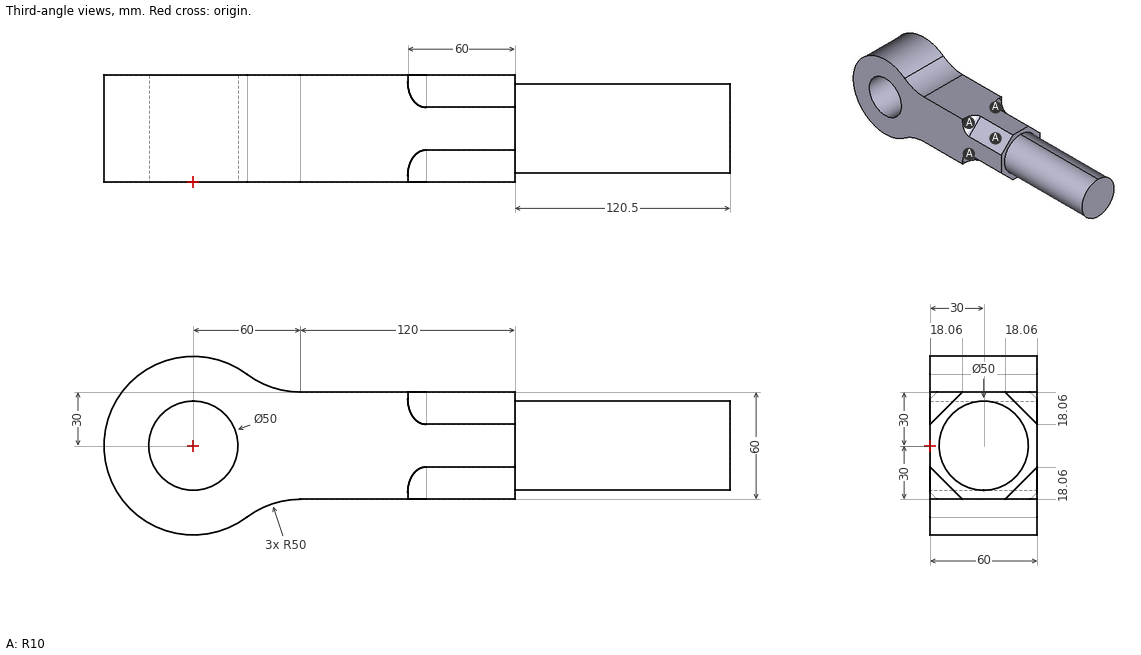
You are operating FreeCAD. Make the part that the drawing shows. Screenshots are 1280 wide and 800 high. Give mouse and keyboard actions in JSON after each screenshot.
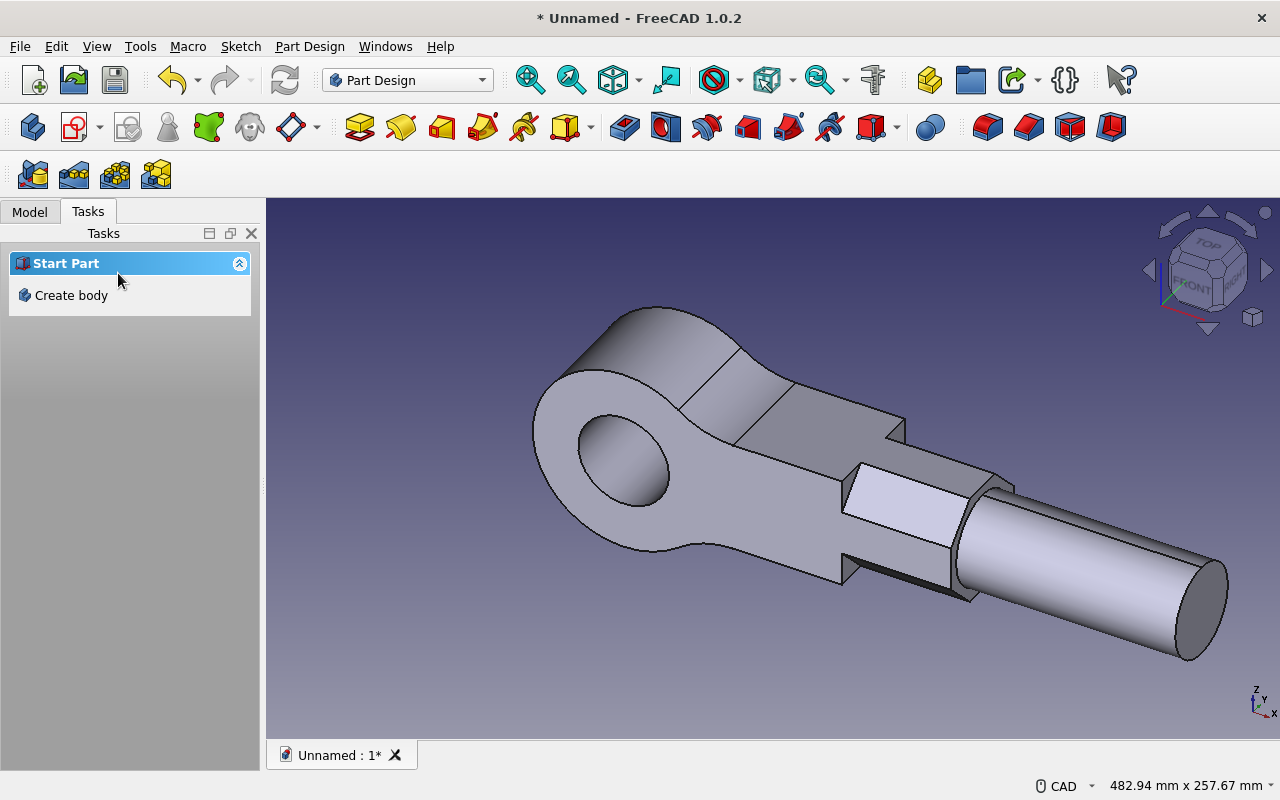
{"action": "key", "text": "0"}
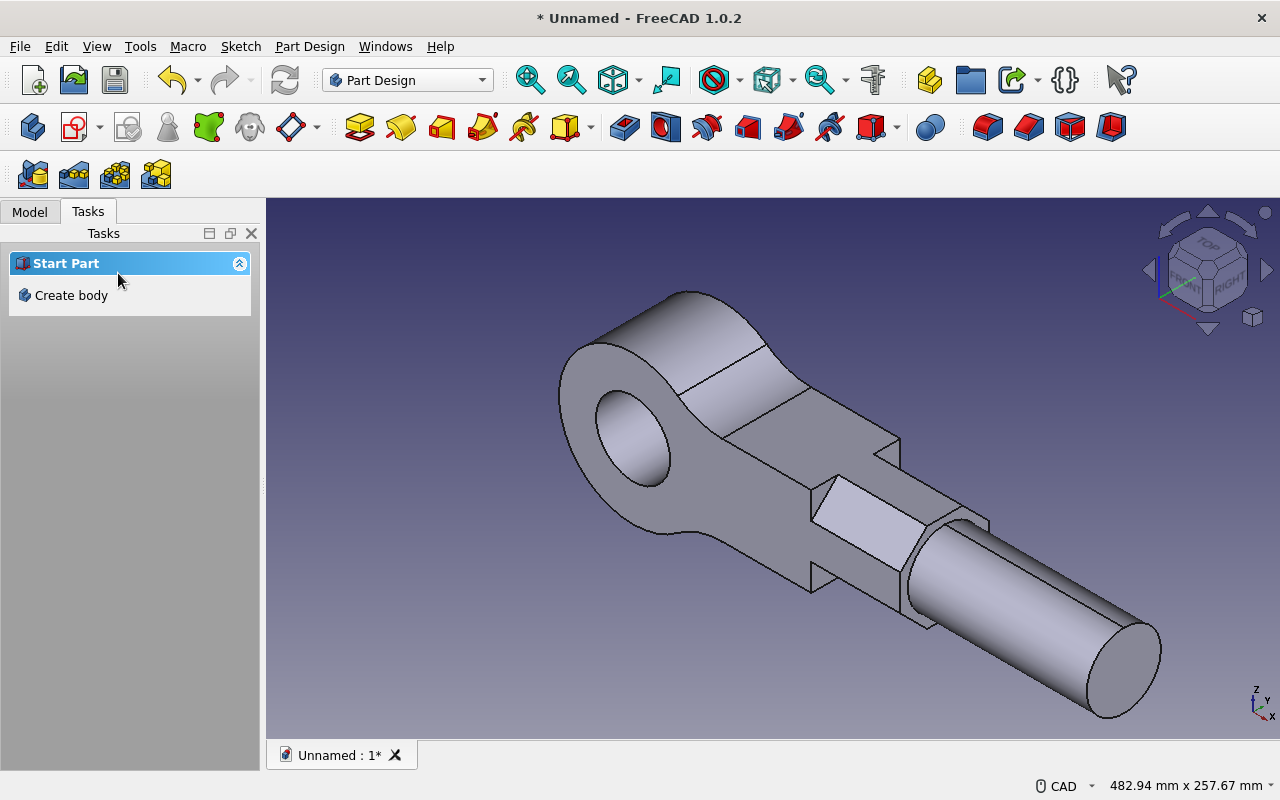
{"action": "key", "text": "v f"}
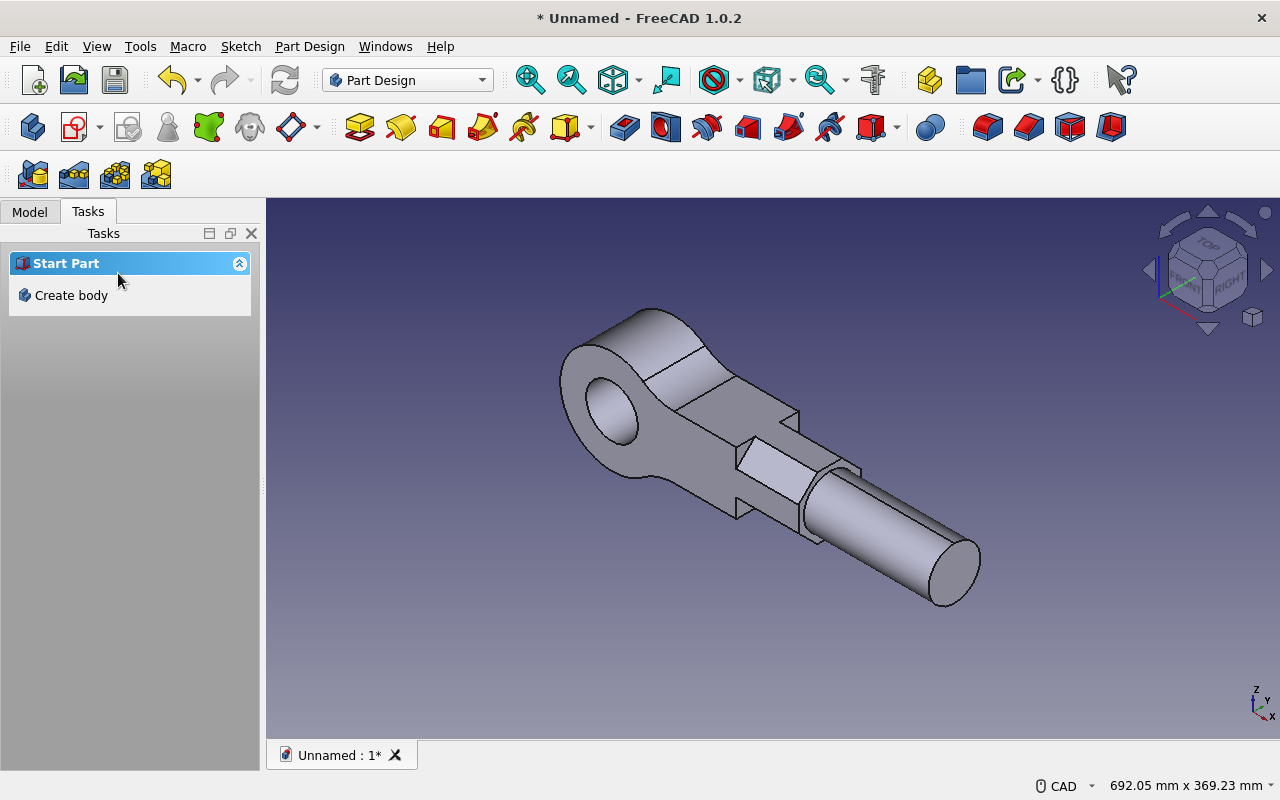
{"action": "key", "text": "2"}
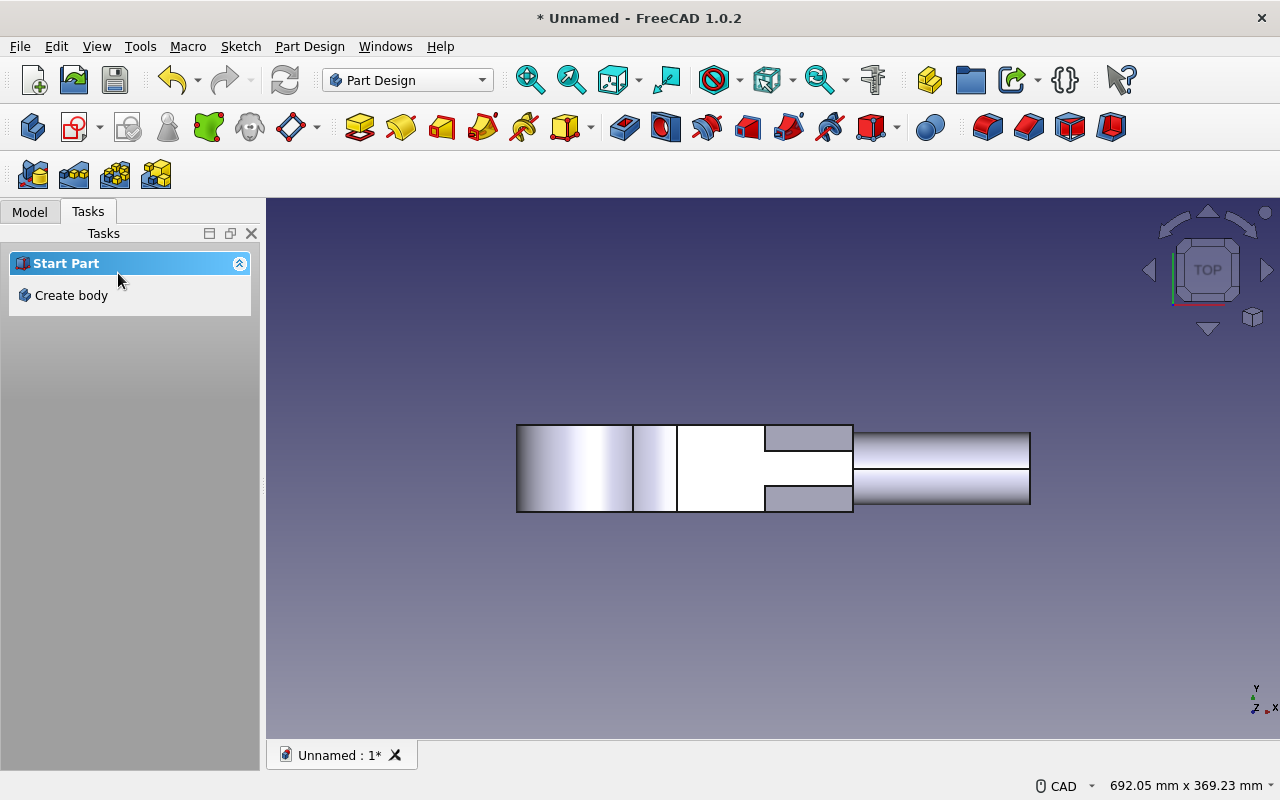
{"action": "key", "text": "1"}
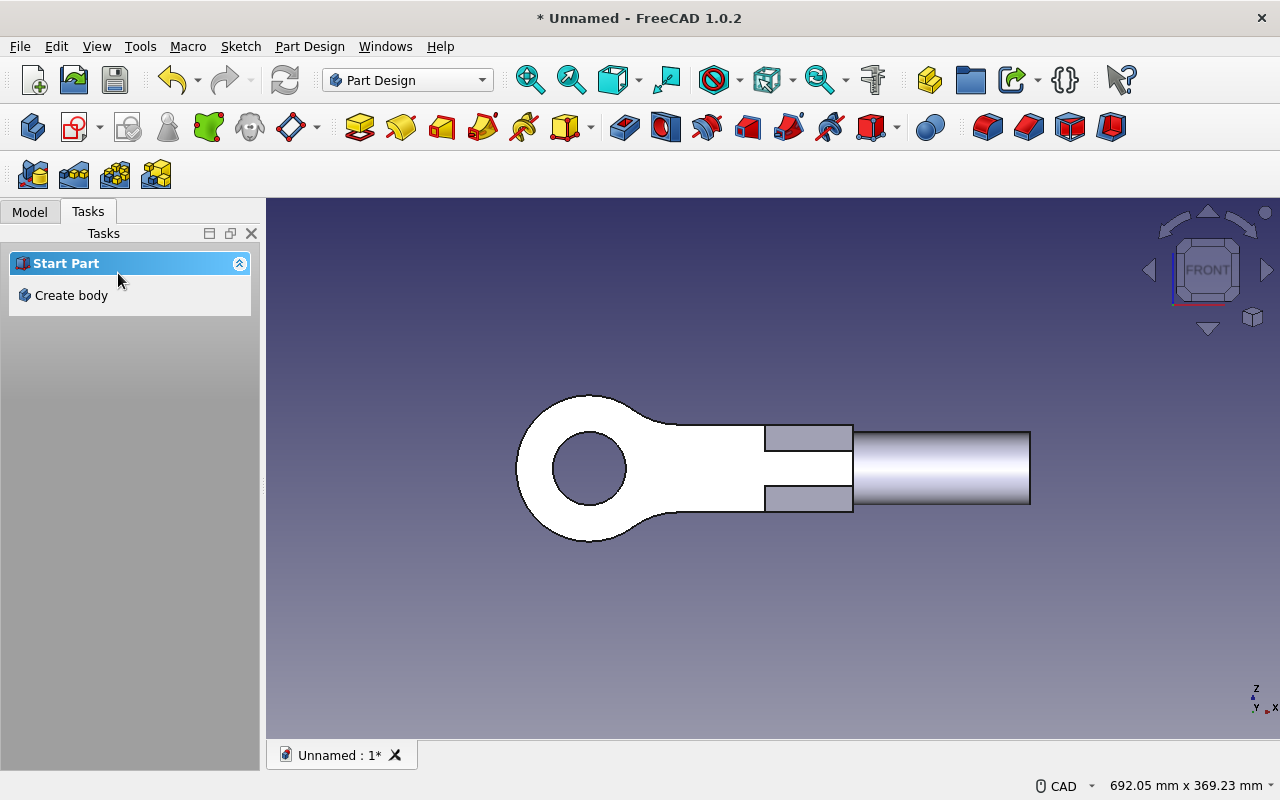
{"action": "key", "text": "3"}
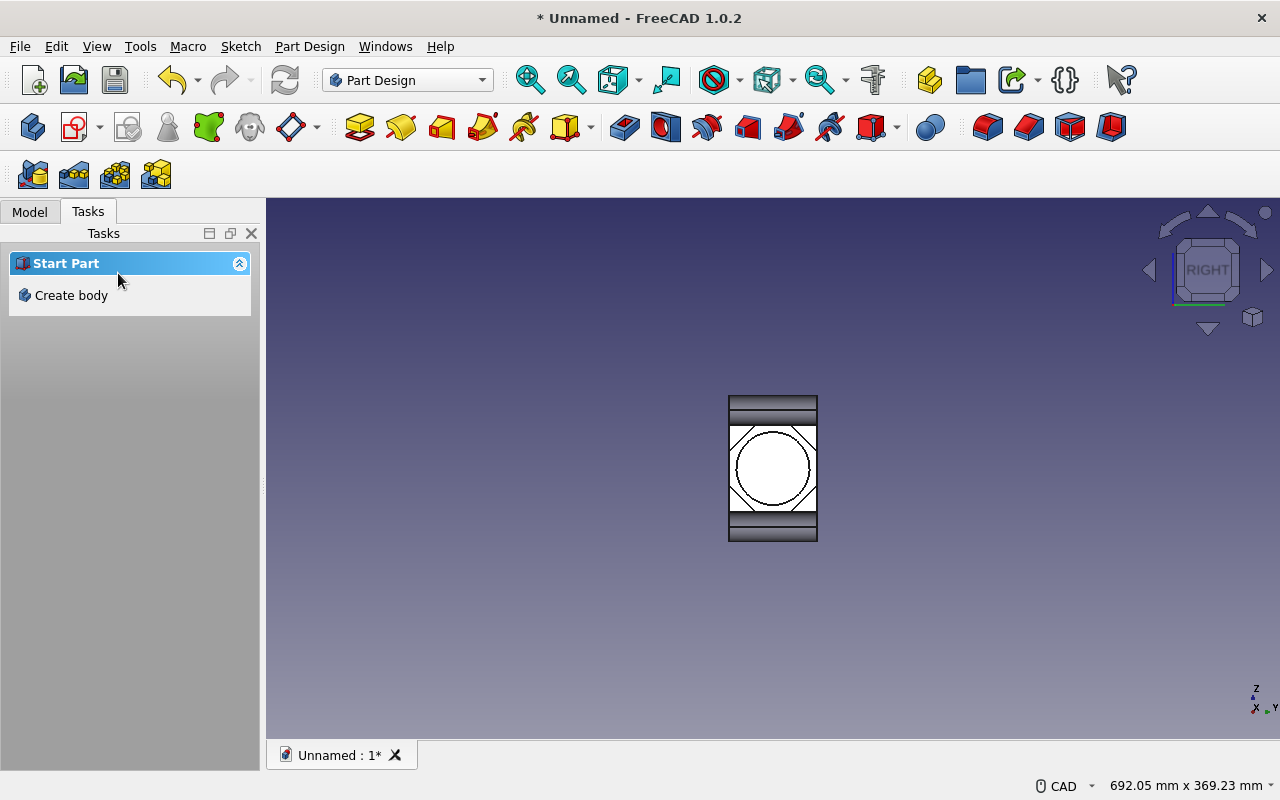
{"action": "key", "text": "v f"}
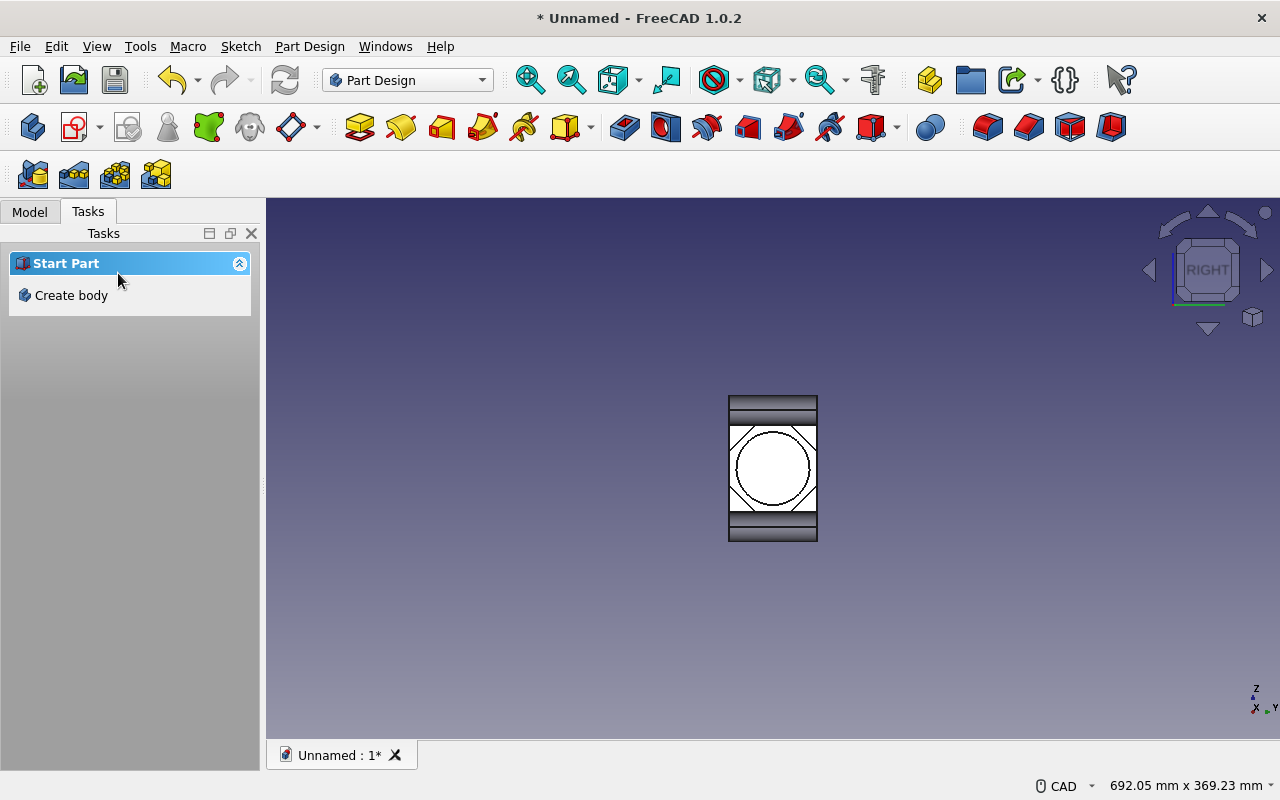
{"action": "key", "text": "5"}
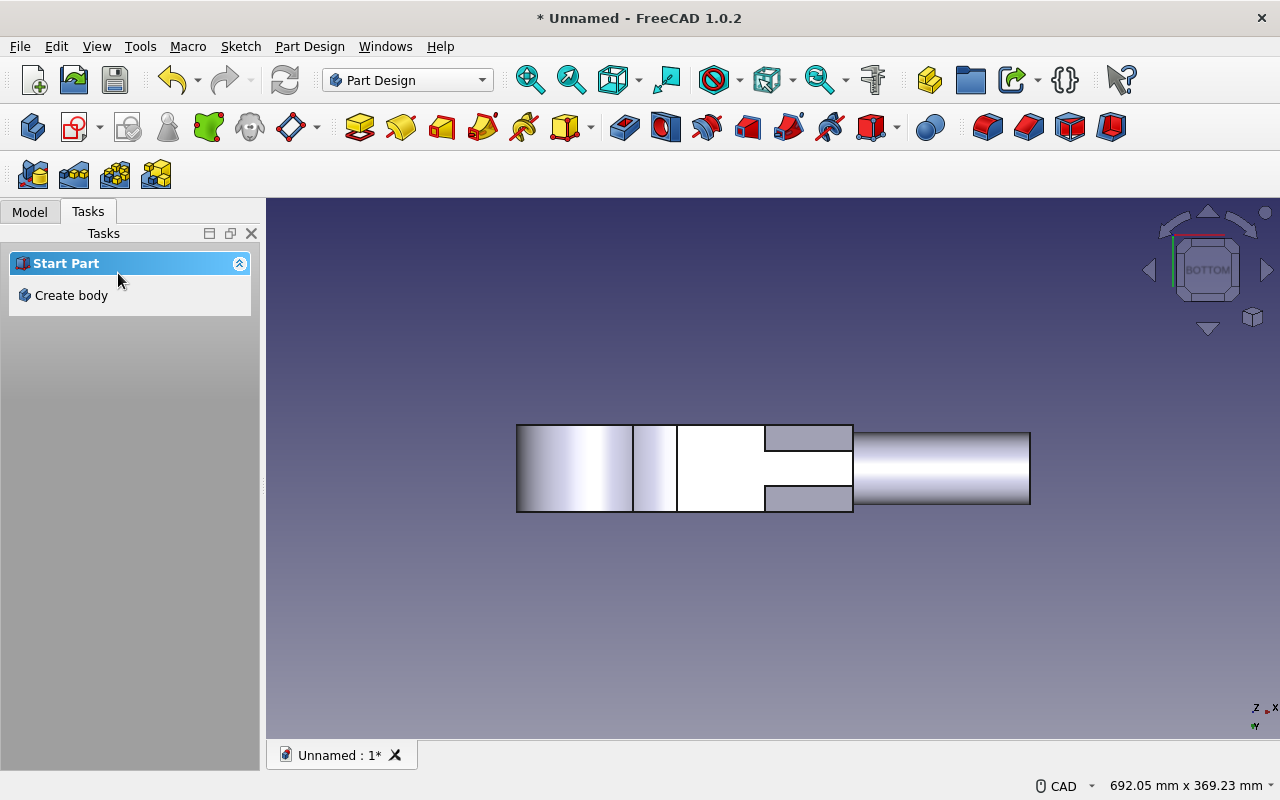
{"action": "key", "text": "4"}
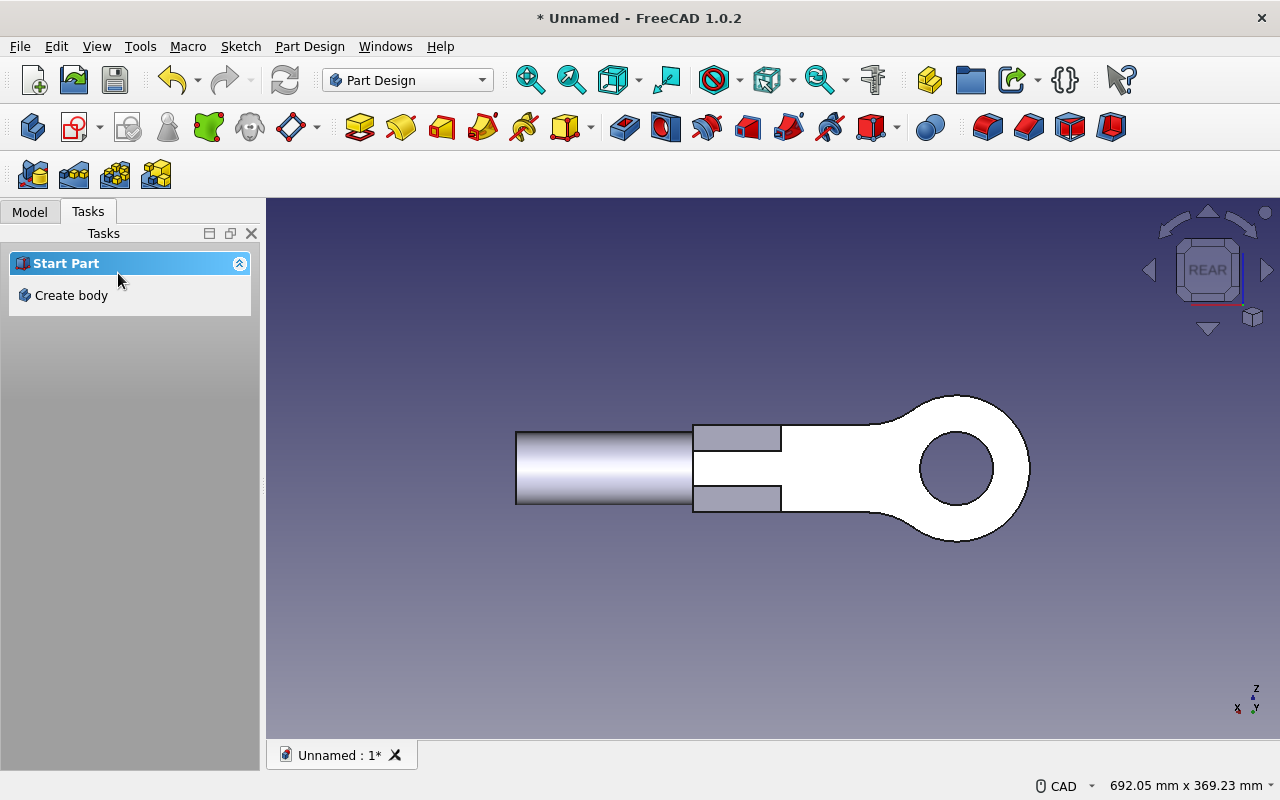
{"action": "key", "text": "6"}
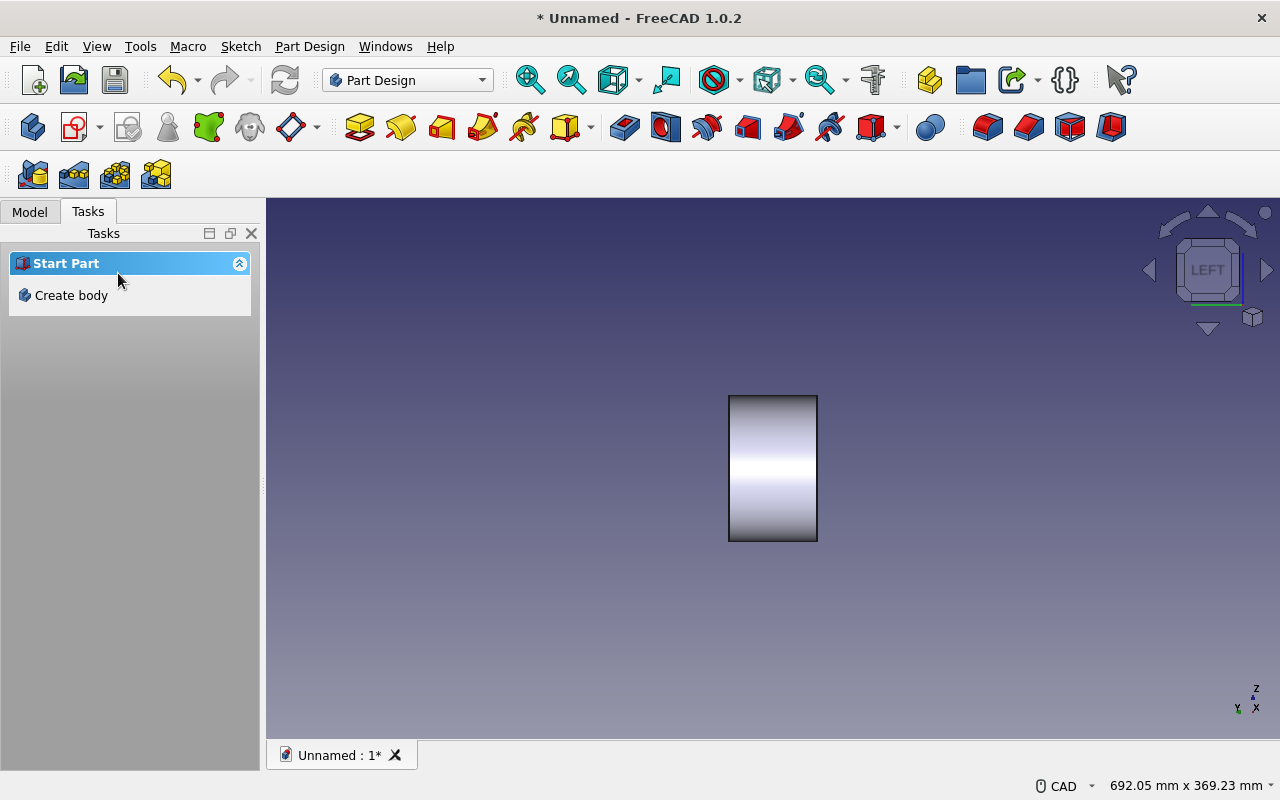
{"action": "left_click", "coordinate": [531, 80]}